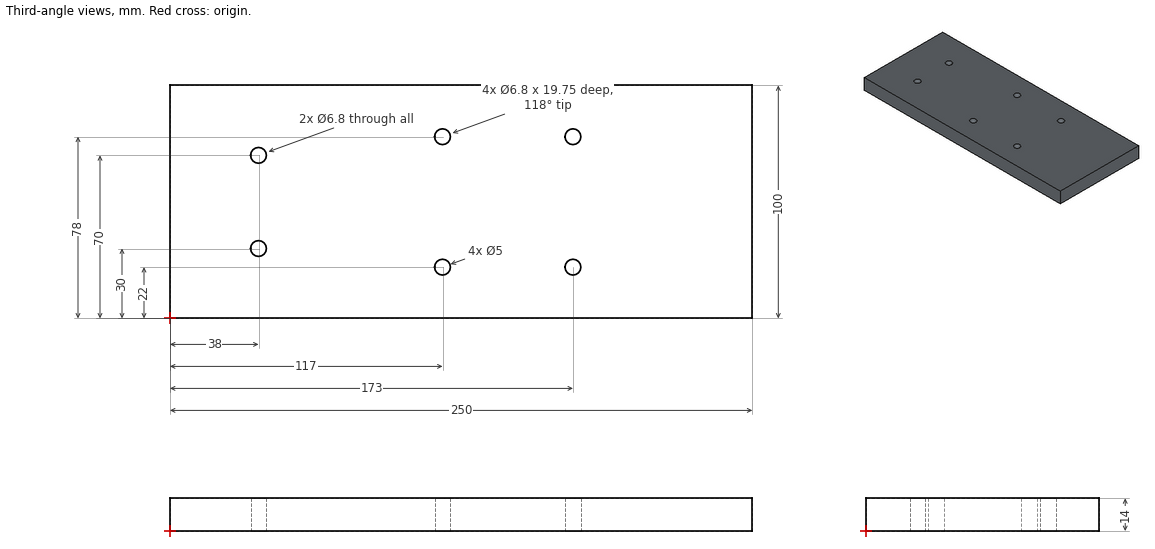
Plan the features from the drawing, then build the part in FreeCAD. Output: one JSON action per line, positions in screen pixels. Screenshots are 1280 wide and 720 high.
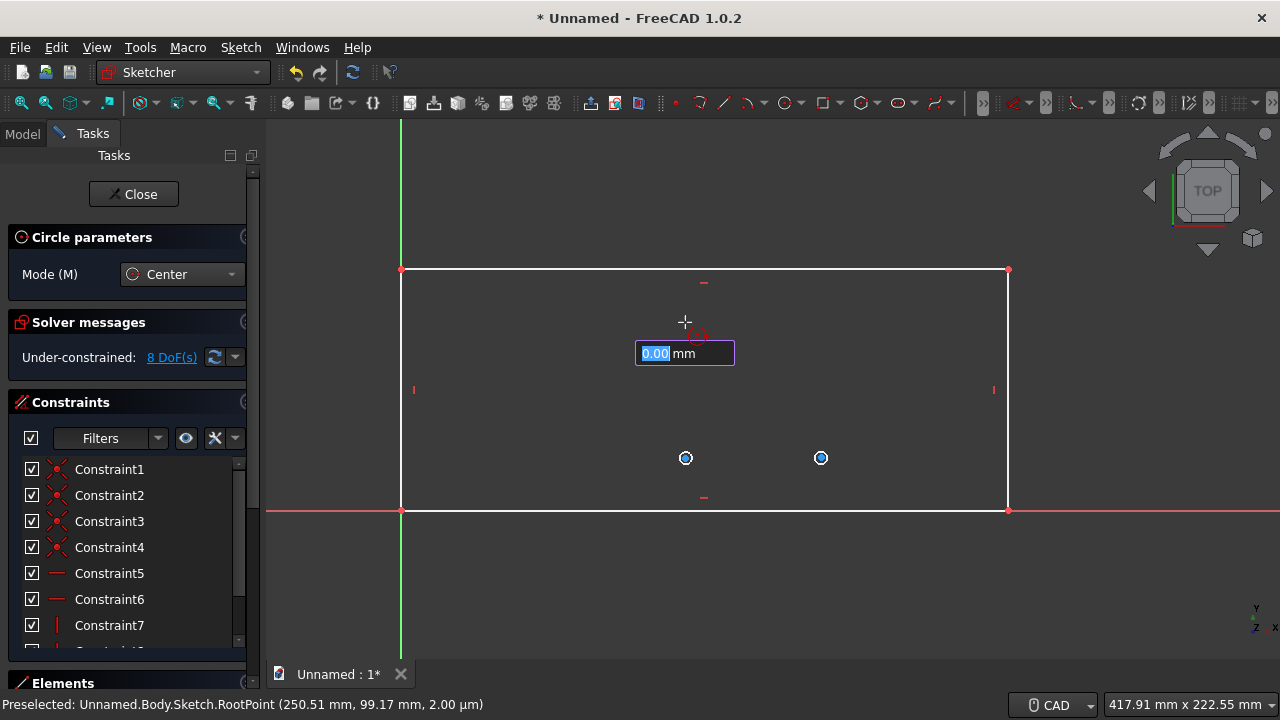
{"action": "scroll", "coordinate": [690, 317], "scroll_direction": "up", "scroll_amount": 5}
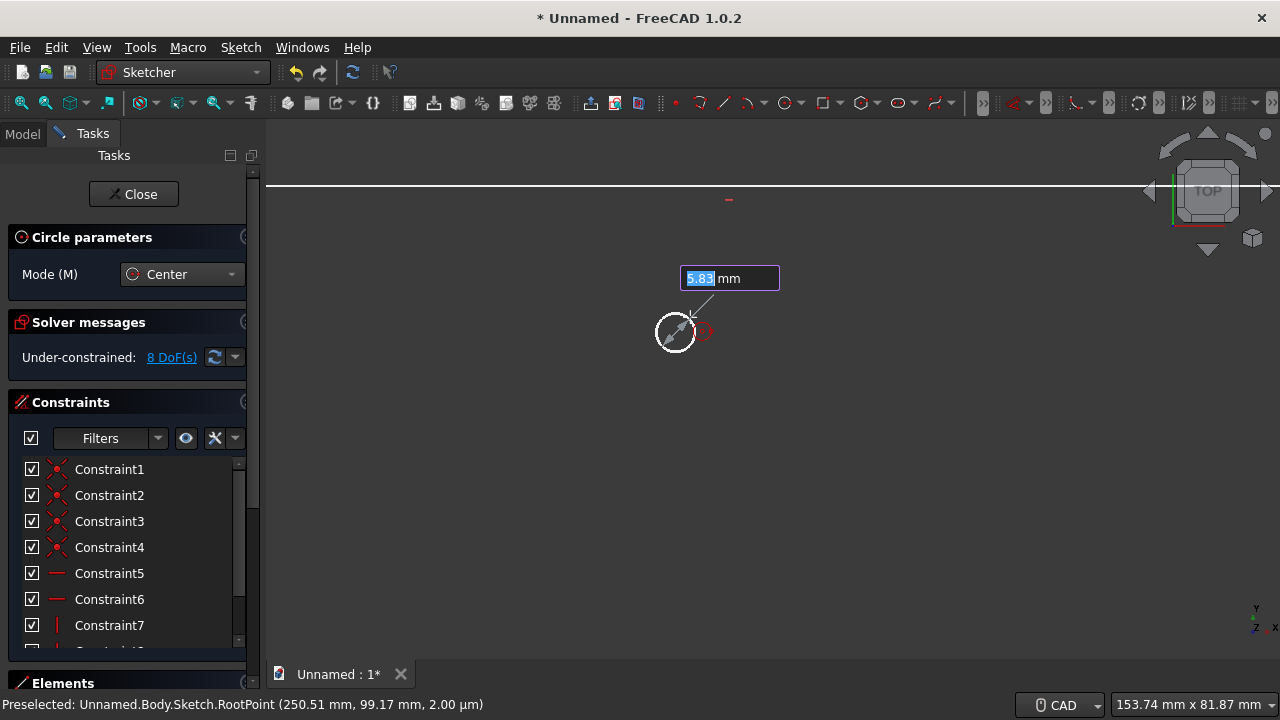
{"action": "left_click", "coordinate": [688, 317]}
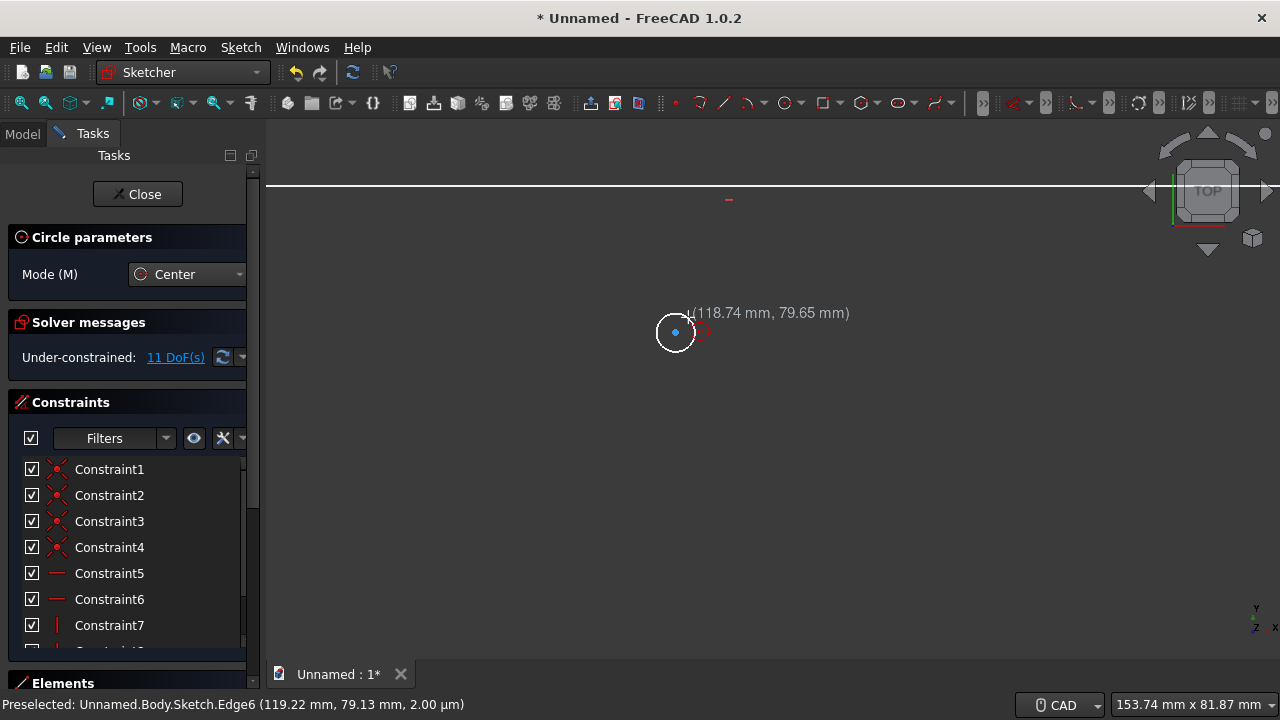
{"action": "scroll", "coordinate": [1046, 329], "scroll_direction": "up", "scroll_amount": 2}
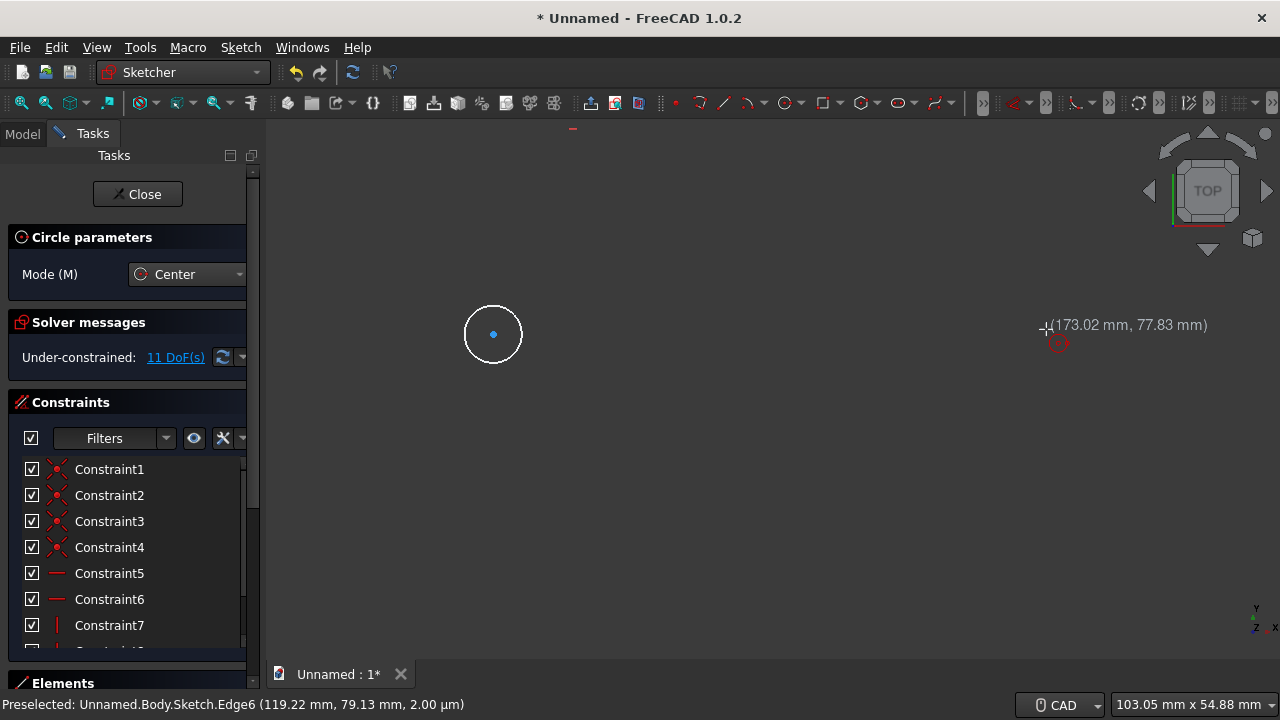
{"action": "scroll", "coordinate": [748, 319], "scroll_direction": "down", "scroll_amount": 7}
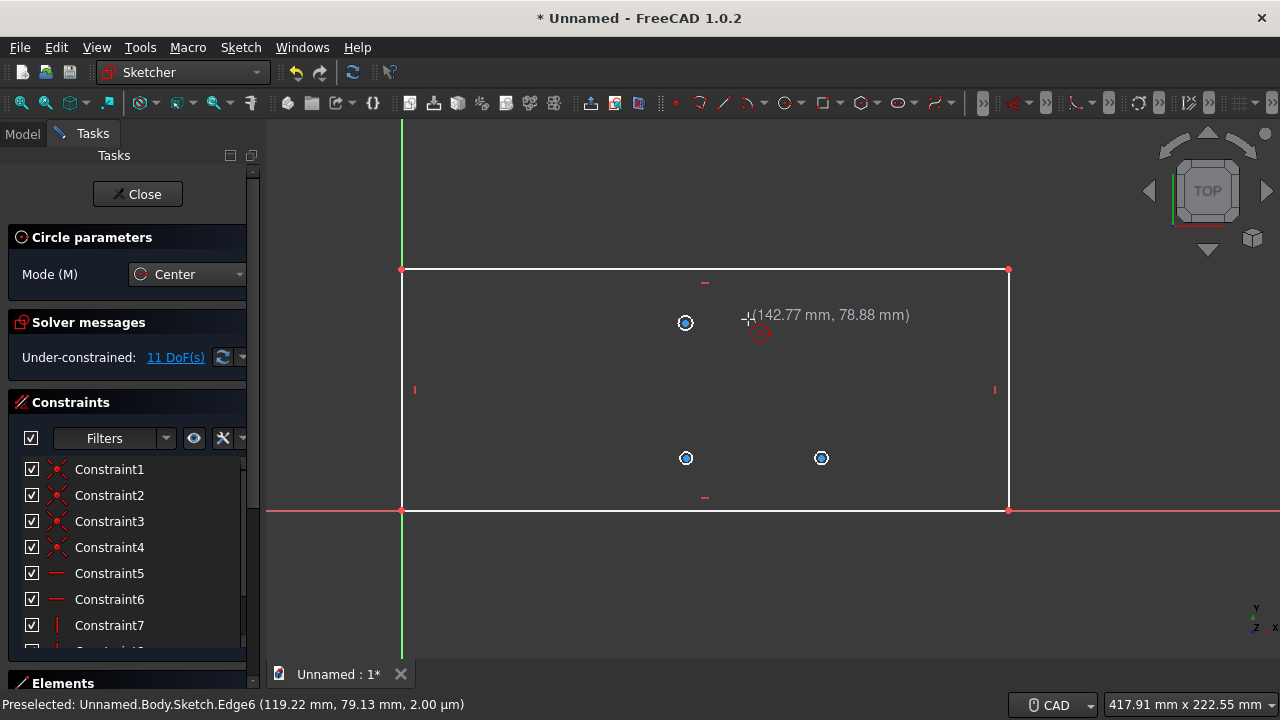
{"action": "left_click", "coordinate": [822, 322]}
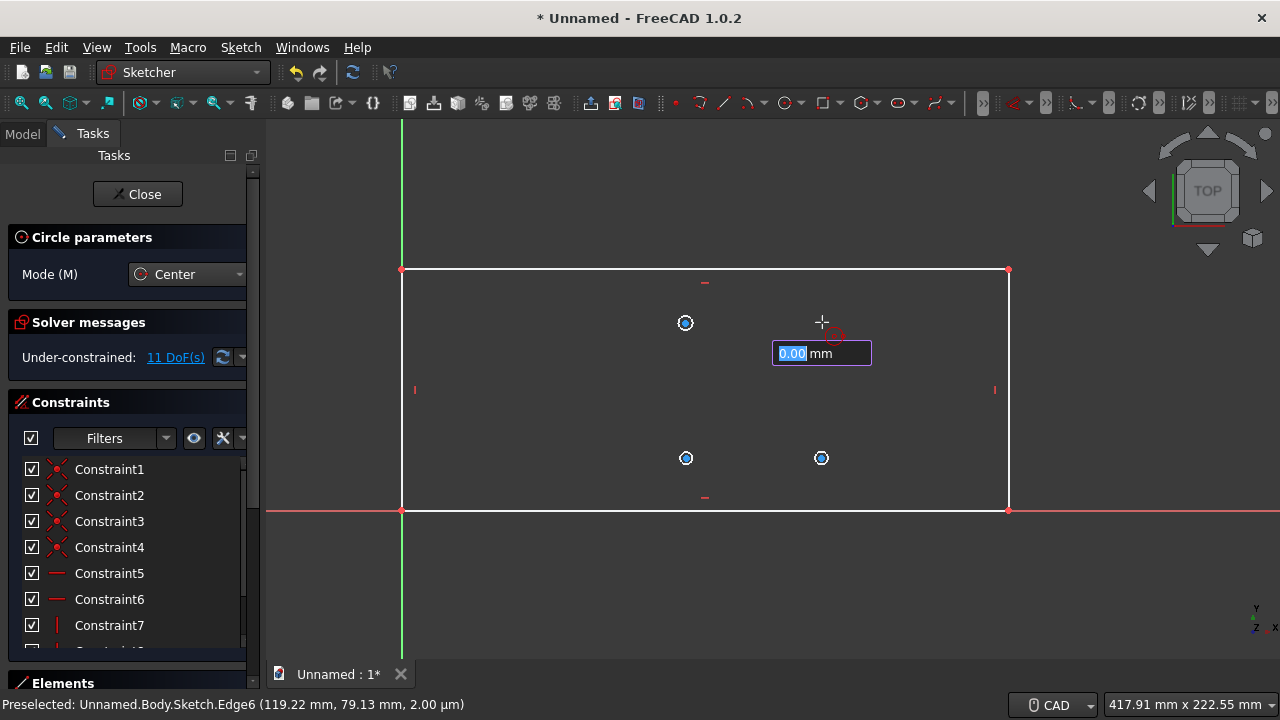
{"action": "scroll", "coordinate": [826, 317], "scroll_direction": "up", "scroll_amount": 5}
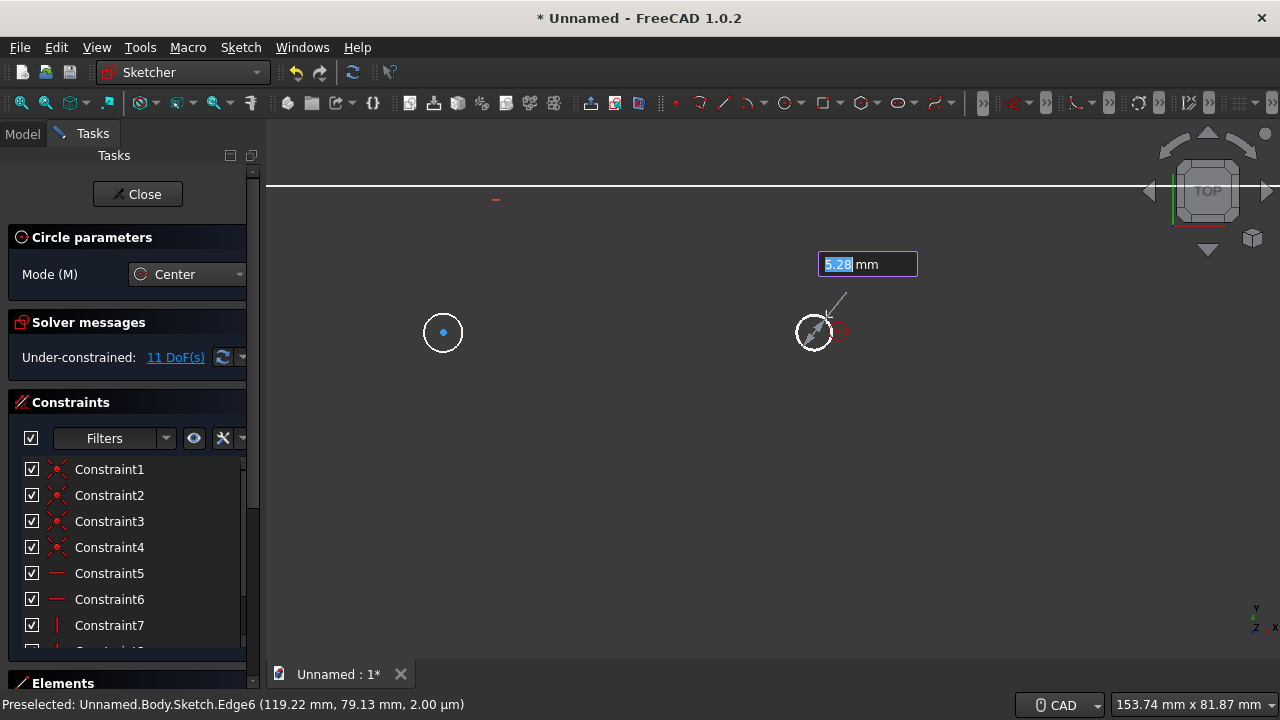
{"action": "left_click", "coordinate": [825, 317]}
{"action": "key", "text": "Escape"}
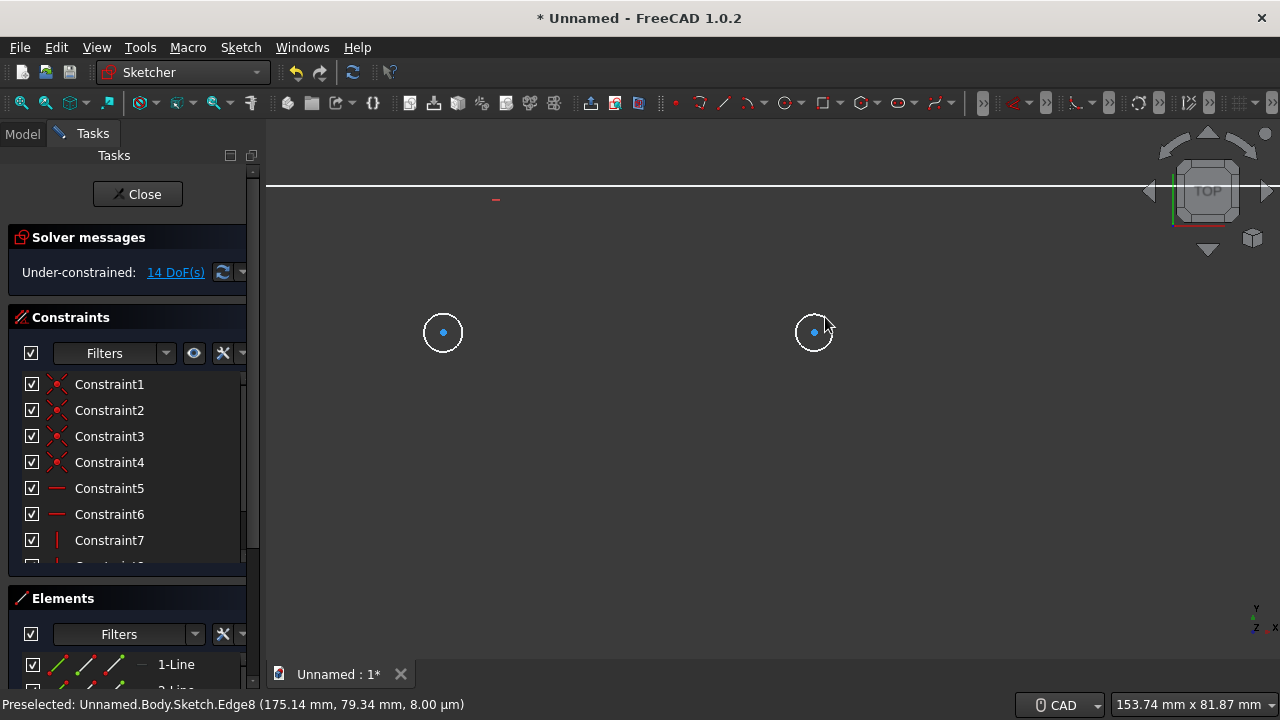
{"action": "scroll", "coordinate": [825, 316], "scroll_direction": "down", "scroll_amount": 5}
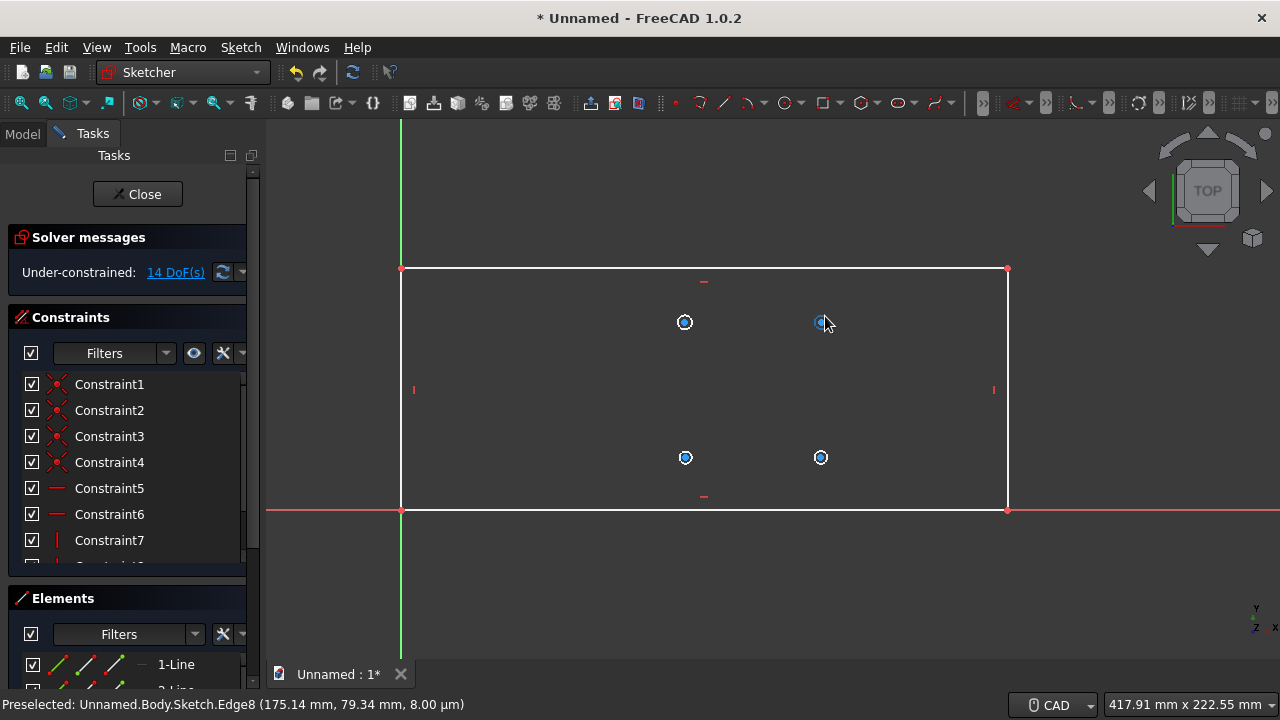
{"action": "scroll", "coordinate": [690, 453], "scroll_direction": "up", "scroll_amount": 5}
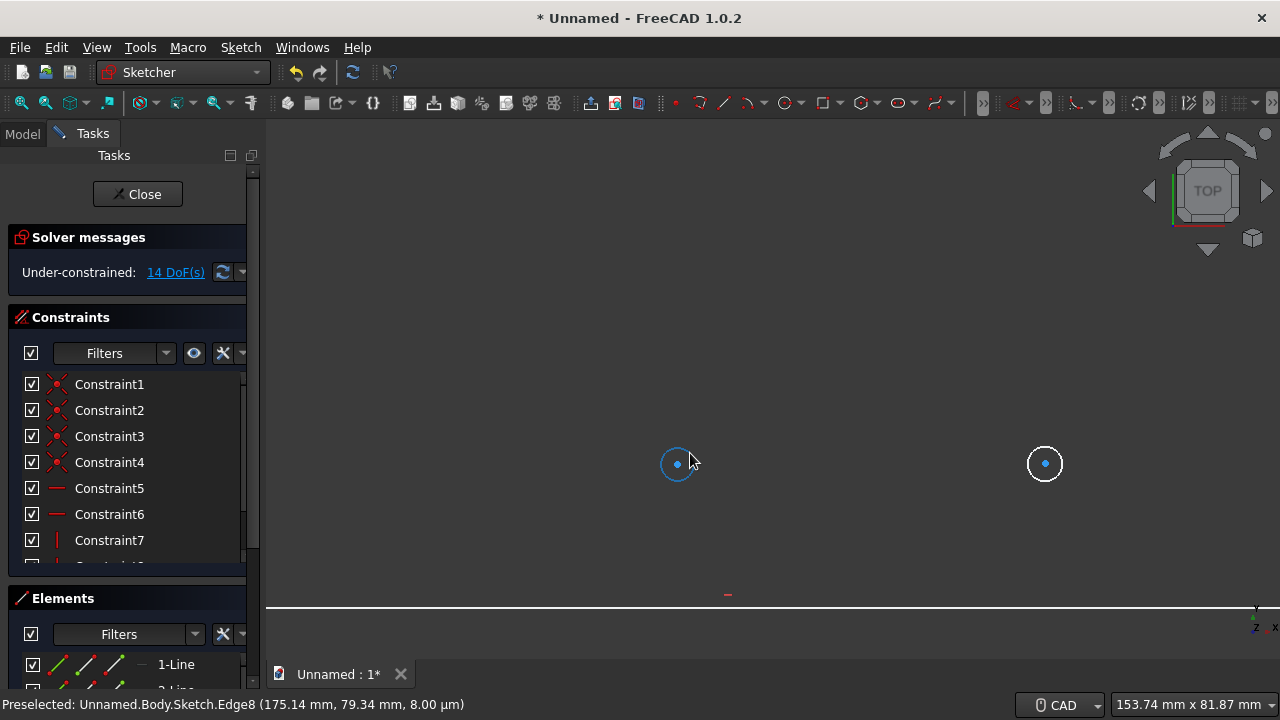
{"action": "left_click", "coordinate": [689, 453]}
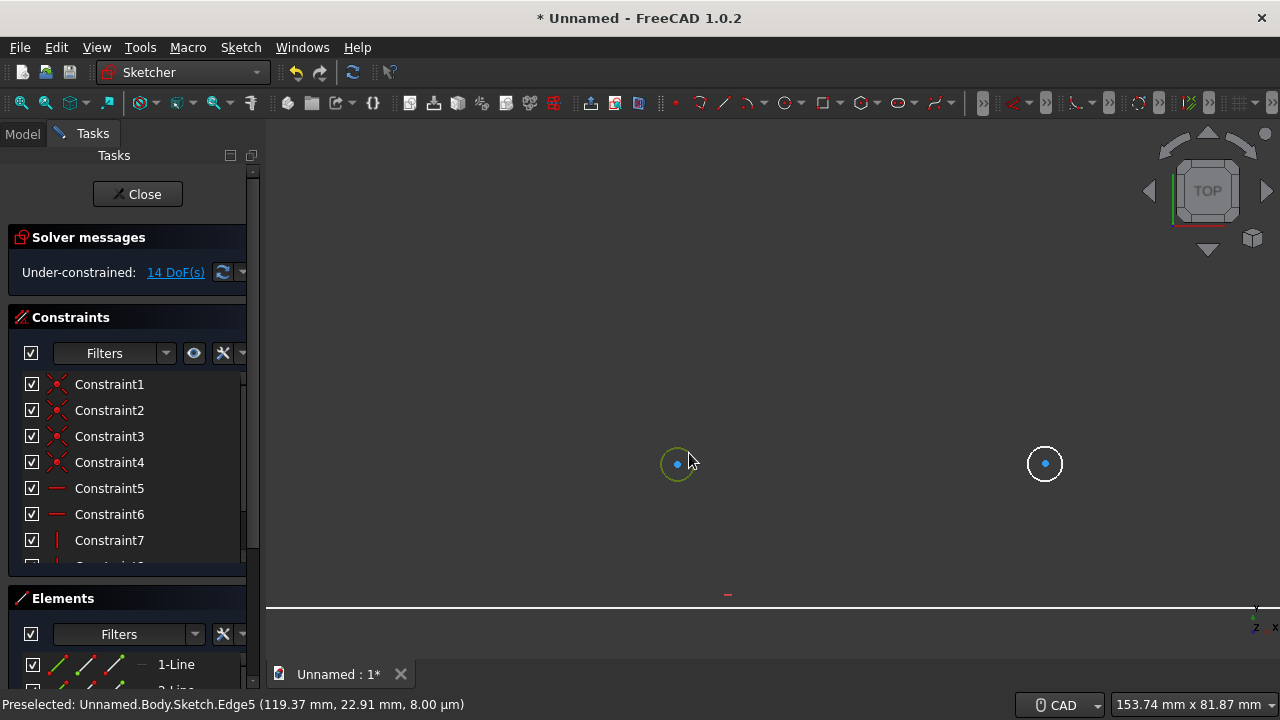
{"action": "left_click", "coordinate": [1057, 452]}